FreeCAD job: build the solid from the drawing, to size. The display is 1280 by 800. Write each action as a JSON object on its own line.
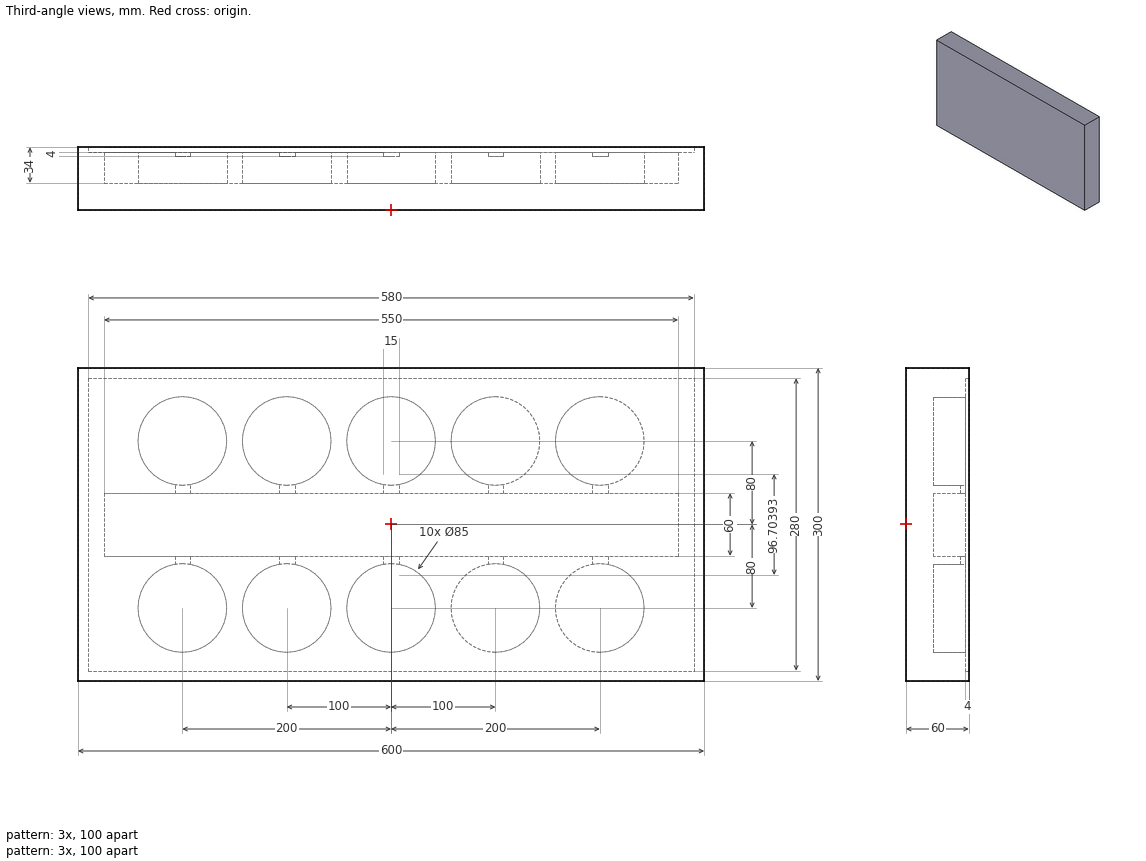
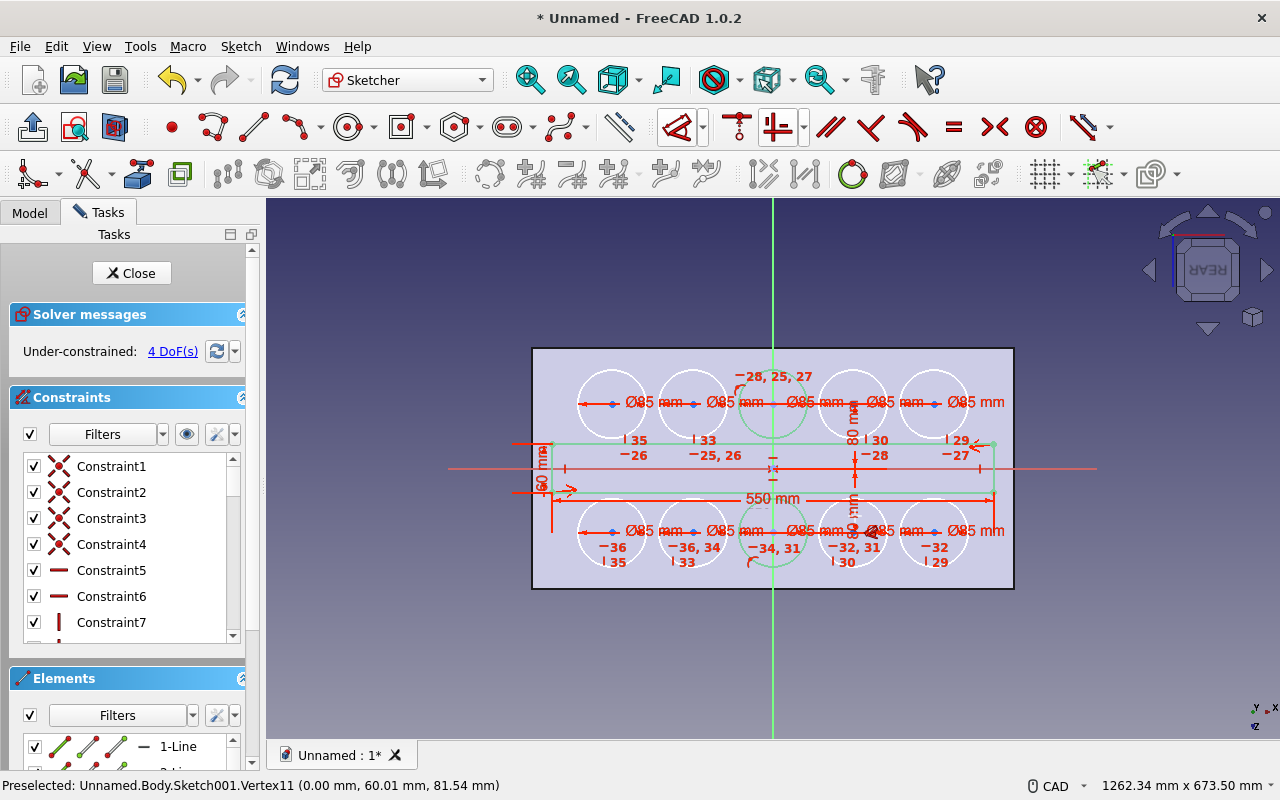
{"action": "left_click", "coordinate": [693, 404]}
{"action": "left_click", "coordinate": [733, 370]}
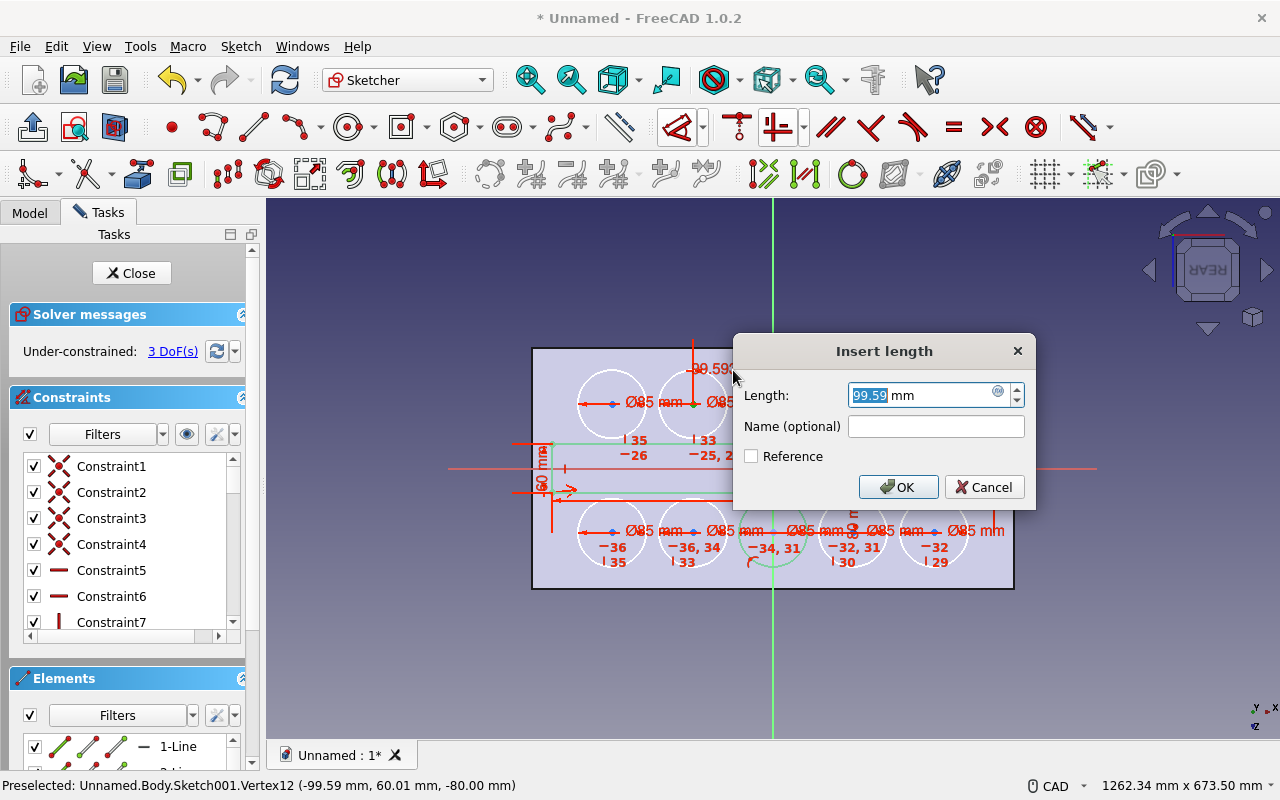
{"action": "type", "text": "100"}
{"action": "key", "text": "Return"}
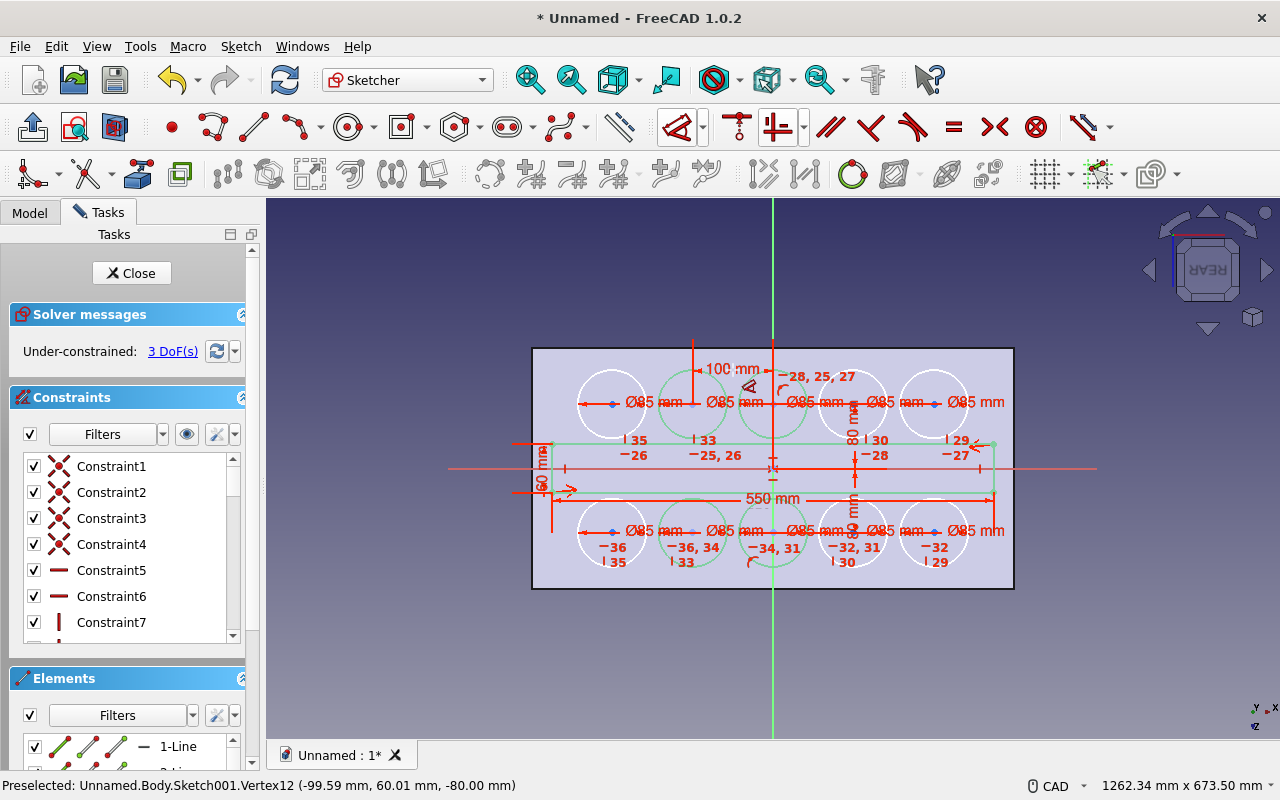
{"action": "left_click", "coordinate": [612, 404]}
{"action": "left_click", "coordinate": [655, 370]}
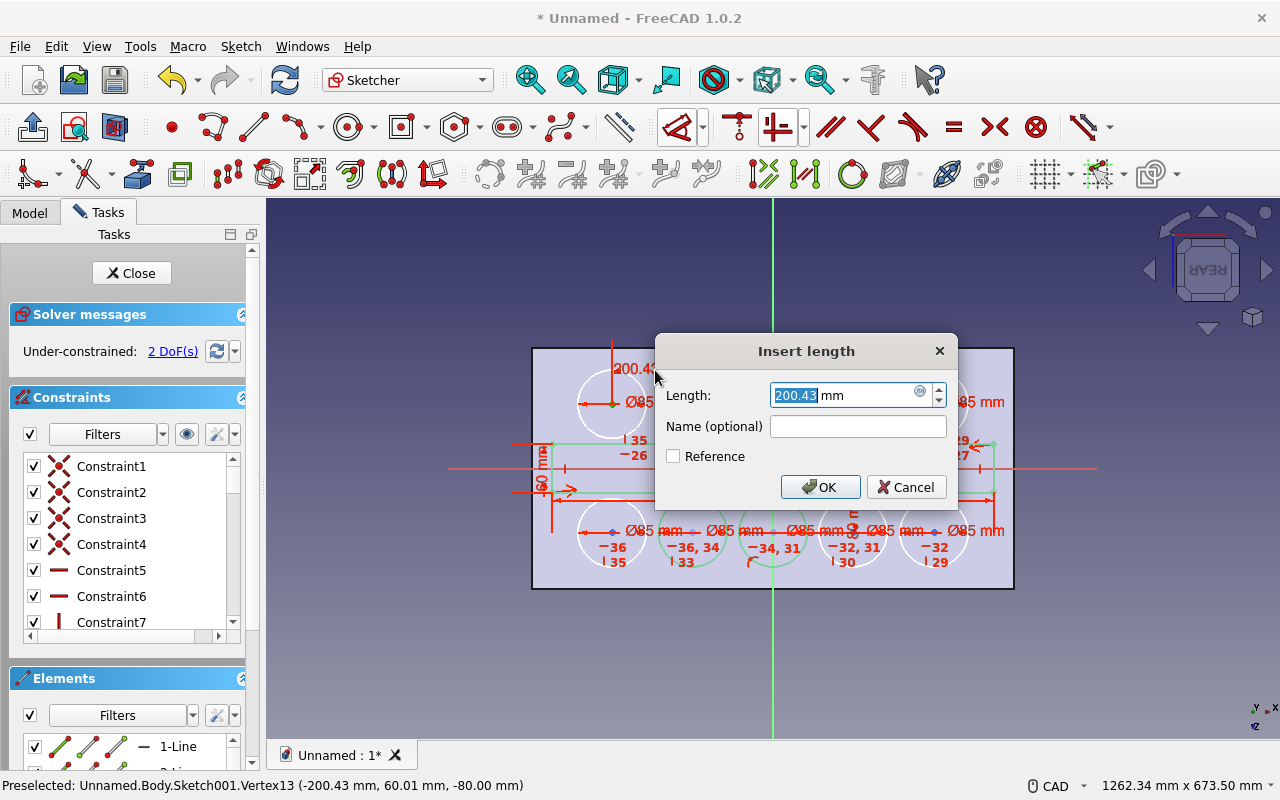
{"action": "type", "text": "200"}
{"action": "key", "text": "Return"}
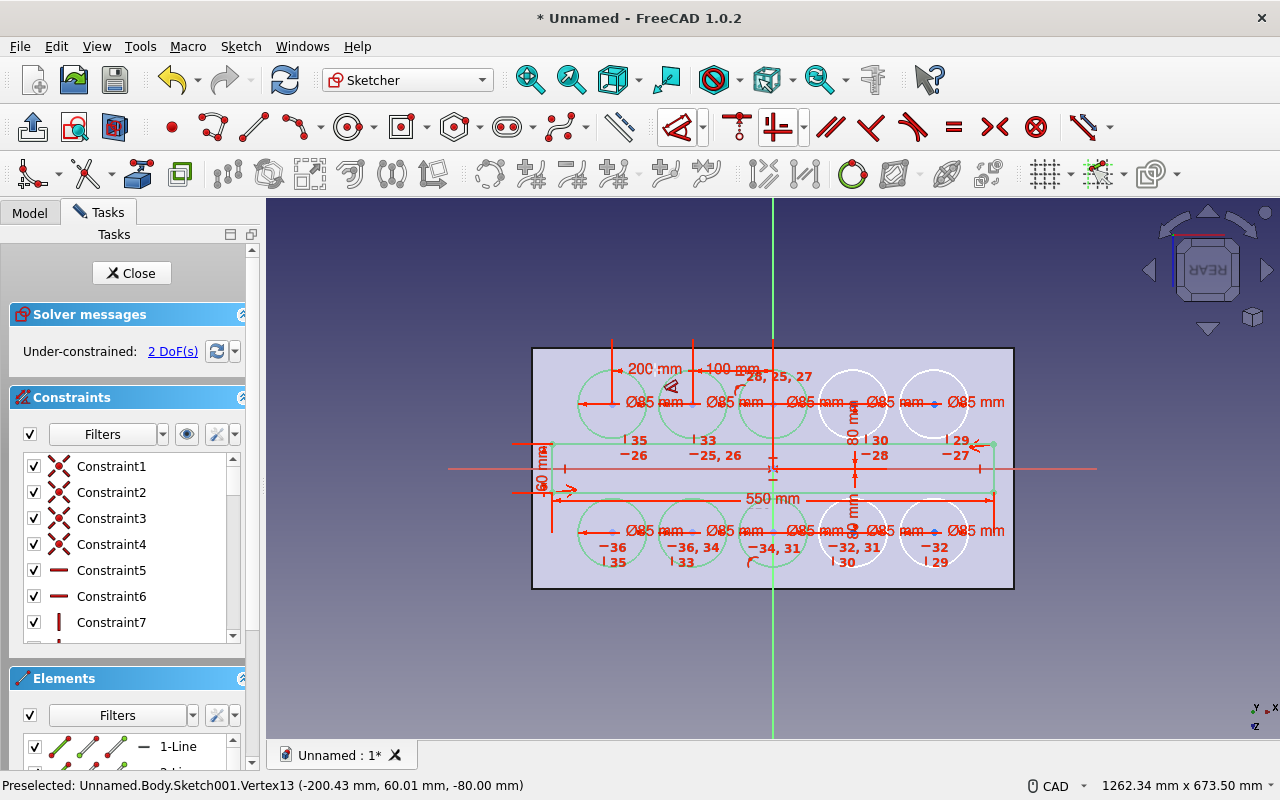
{"action": "left_click", "coordinate": [934, 404]}
{"action": "left_click", "coordinate": [816, 370]}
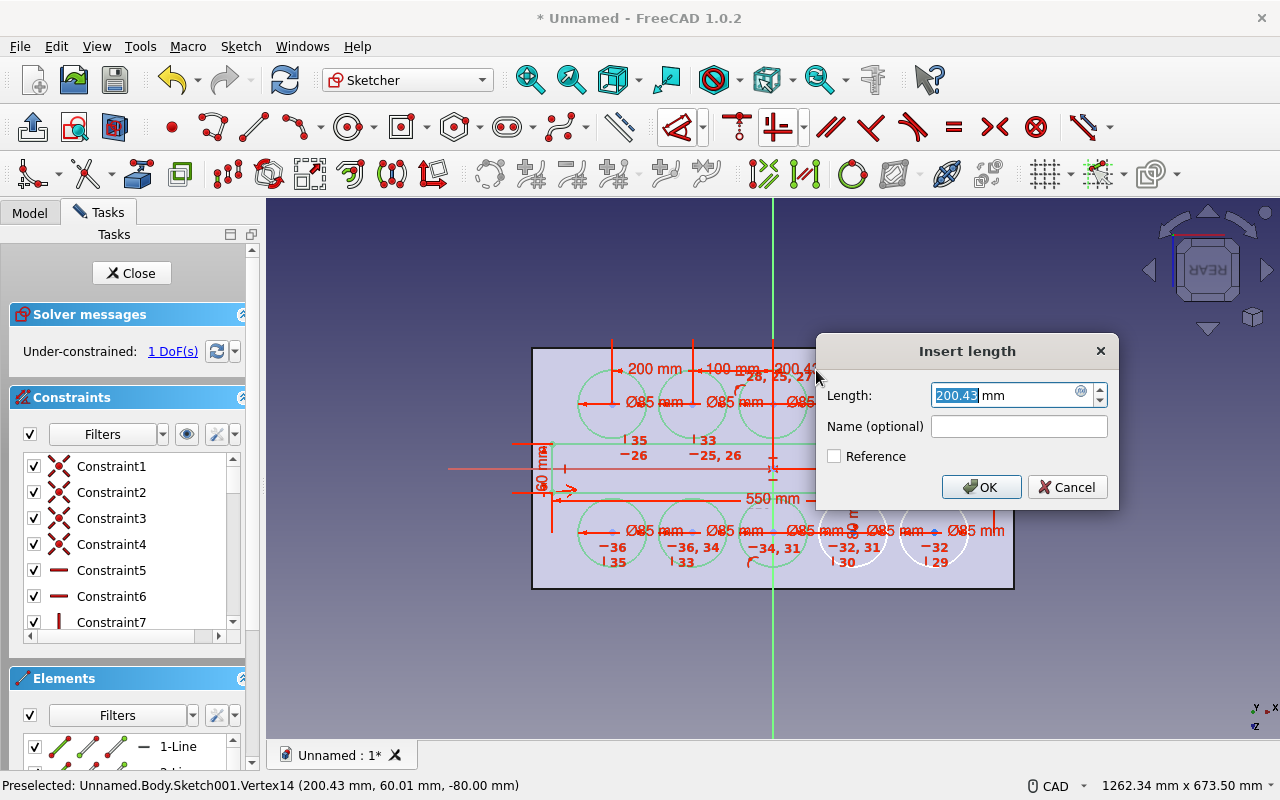
{"action": "type", "text": "200"}
{"action": "key", "text": "Return"}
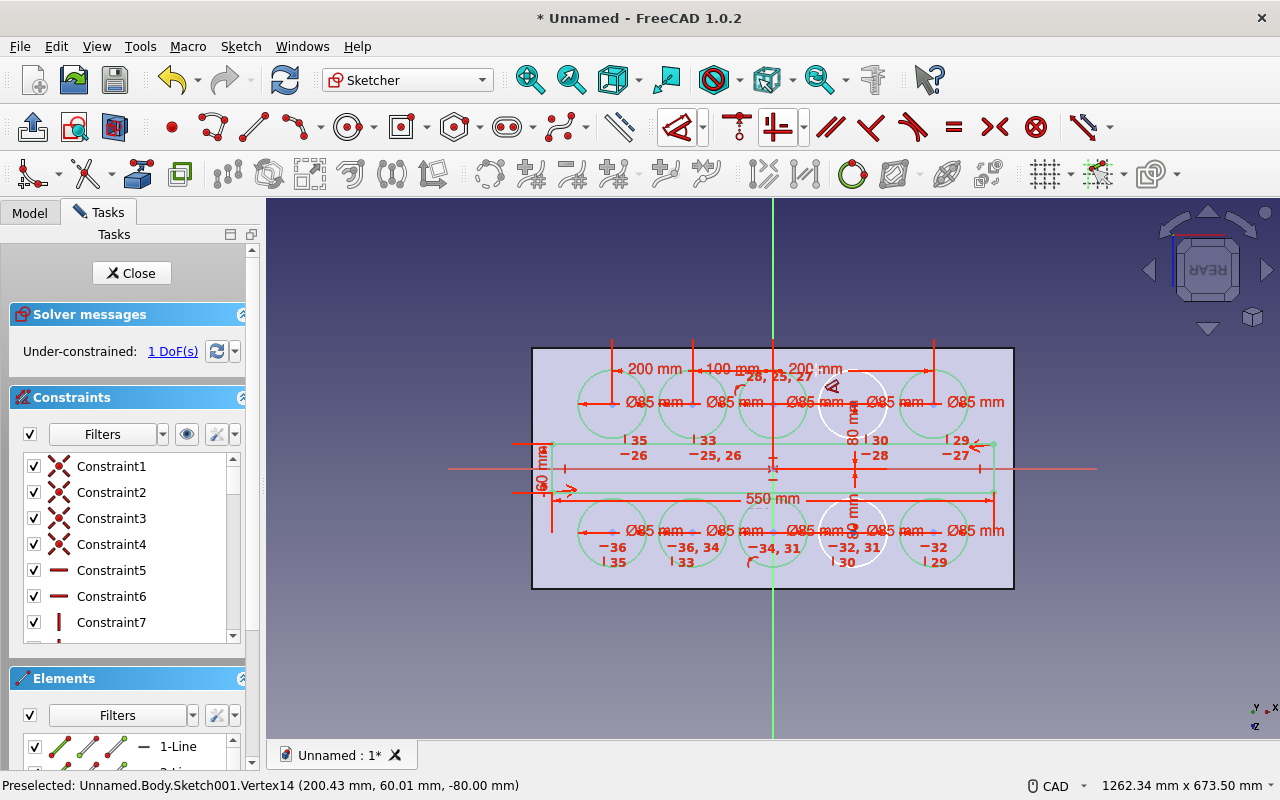
{"action": "left_click", "coordinate": [853, 404]}
{"action": "left_click", "coordinate": [813, 346]}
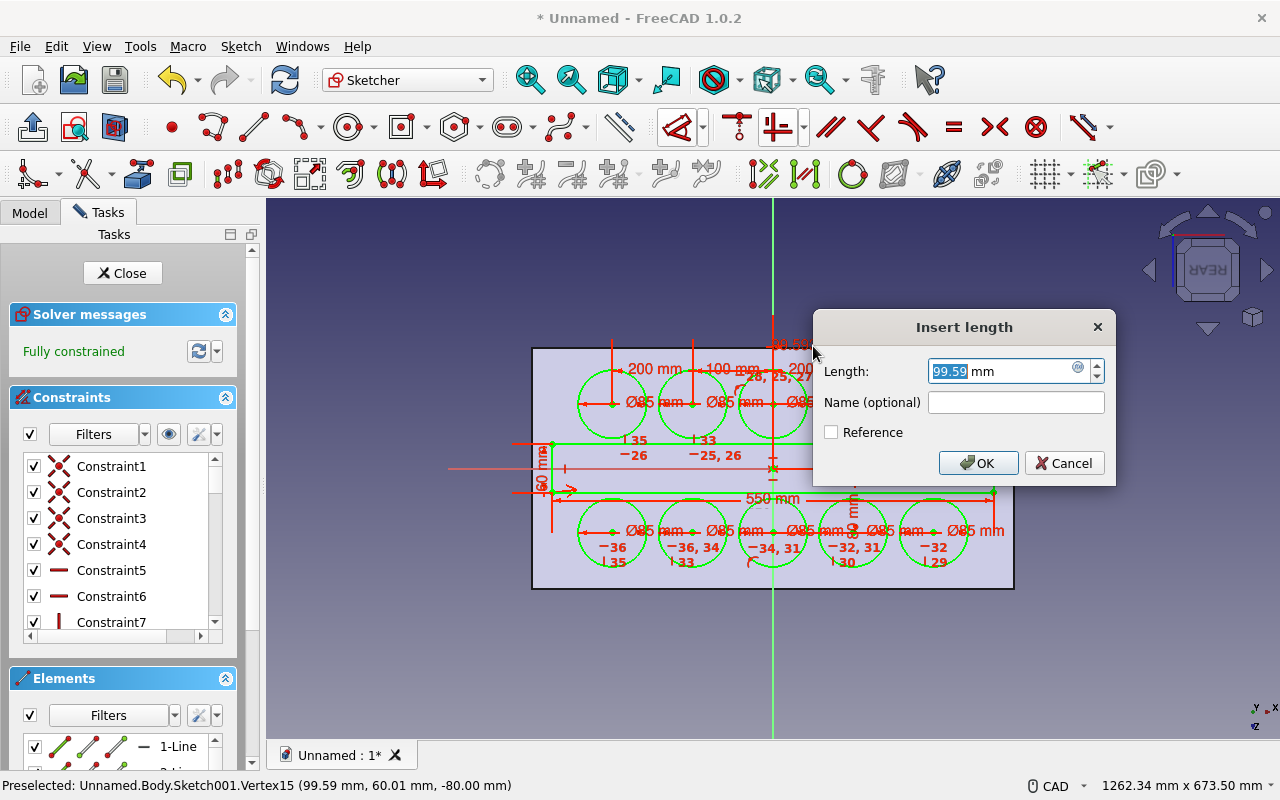
{"action": "type", "text": "100"}
{"action": "key", "text": "Return"}
{"action": "key", "text": "Escape"}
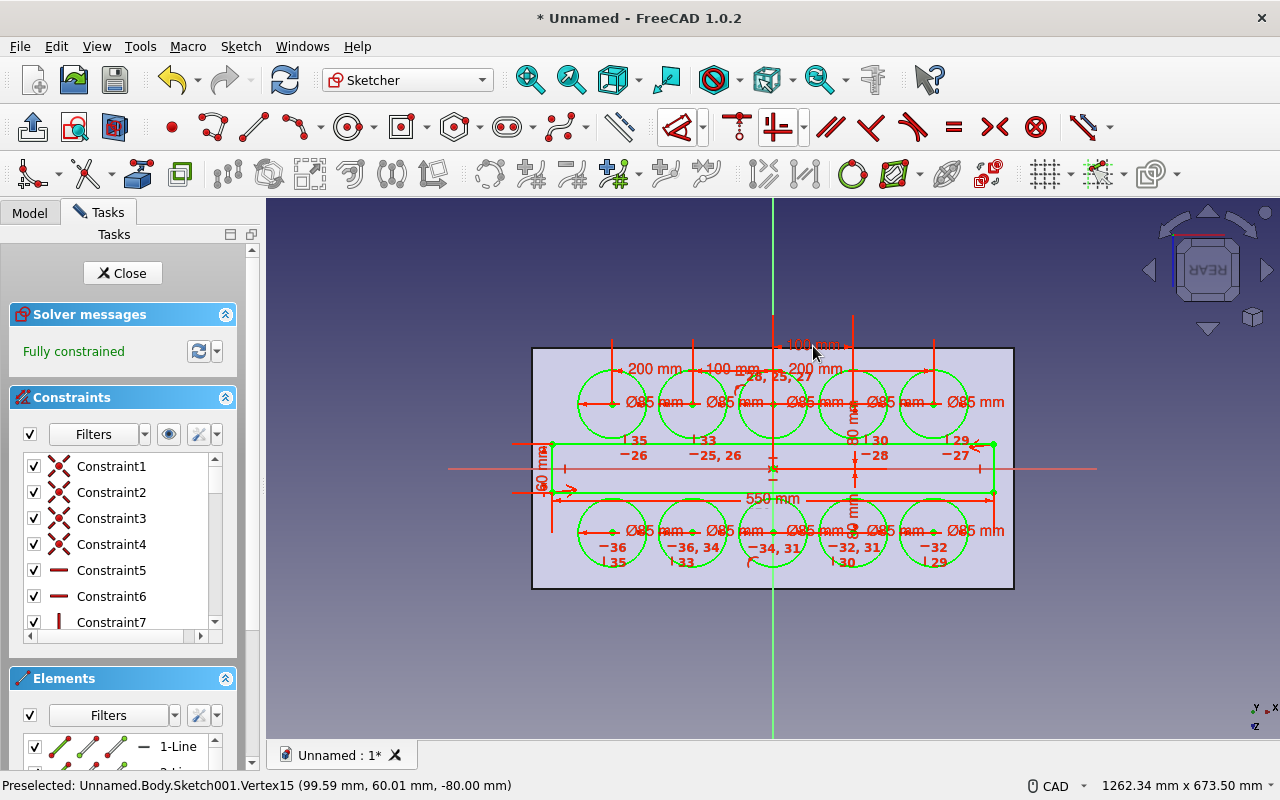
{"action": "left_click", "coordinate": [123, 273]}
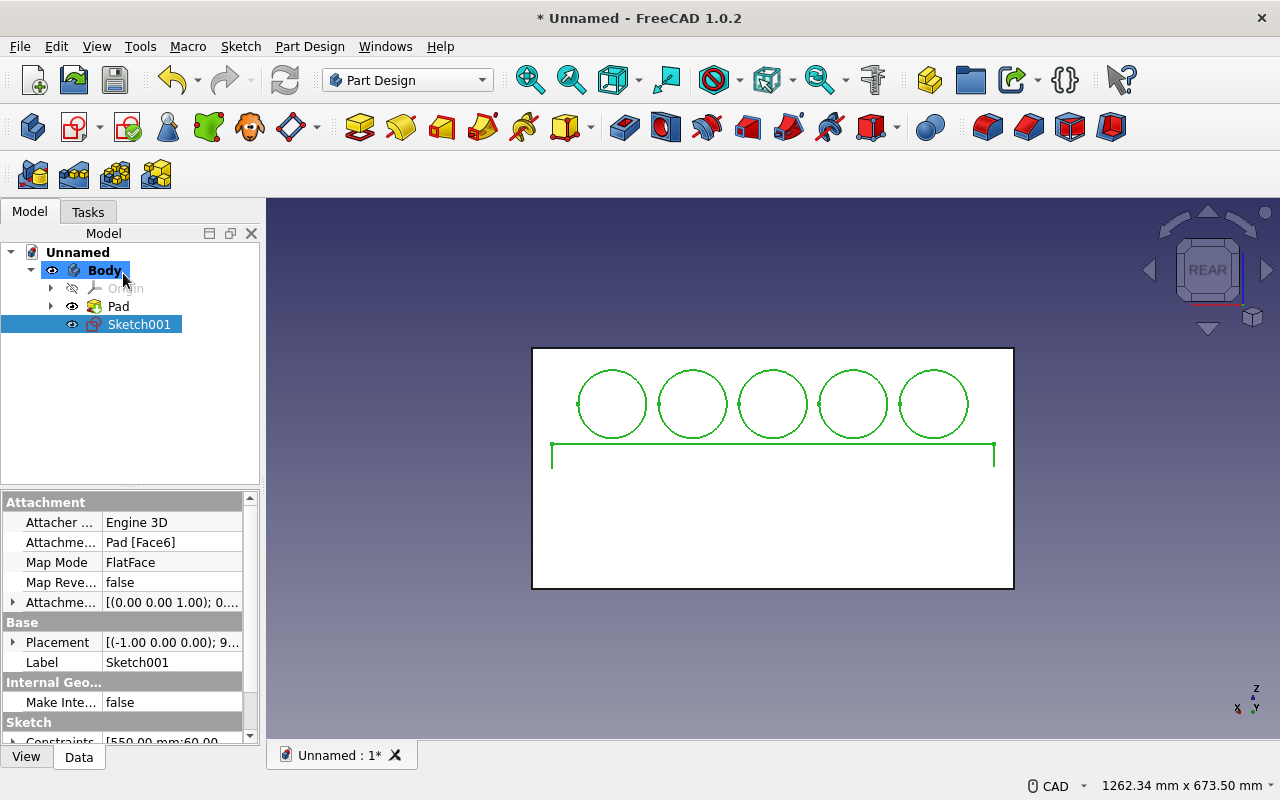
{"action": "left_click", "coordinate": [625, 128]}